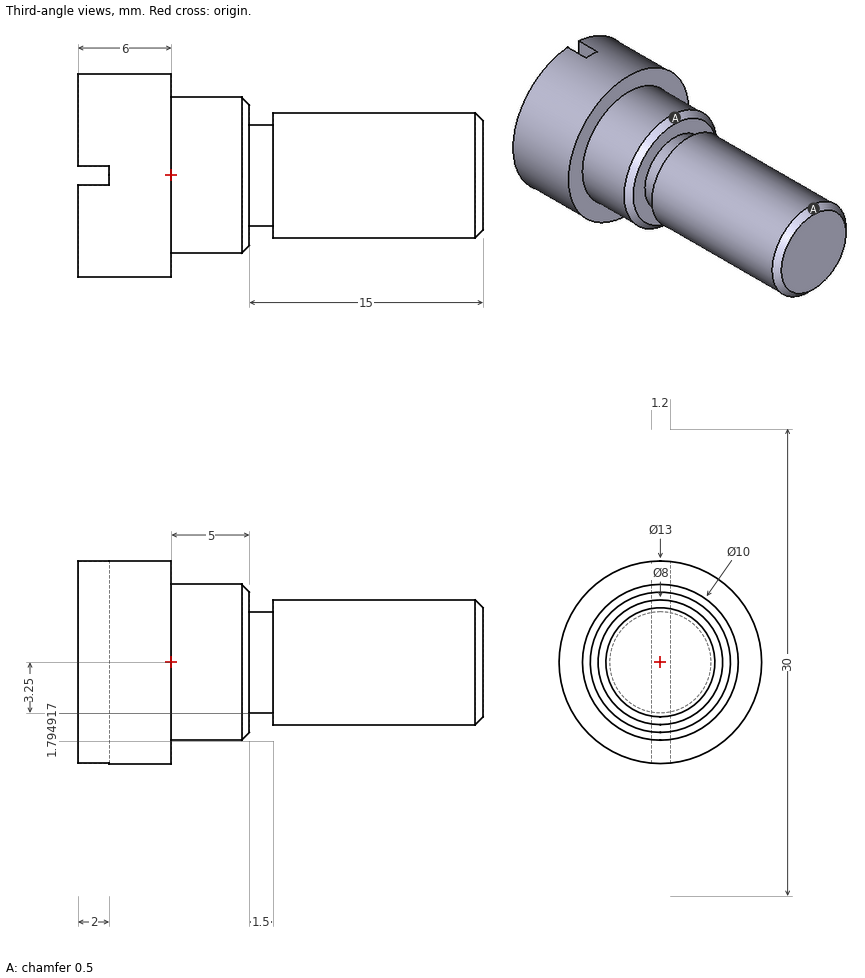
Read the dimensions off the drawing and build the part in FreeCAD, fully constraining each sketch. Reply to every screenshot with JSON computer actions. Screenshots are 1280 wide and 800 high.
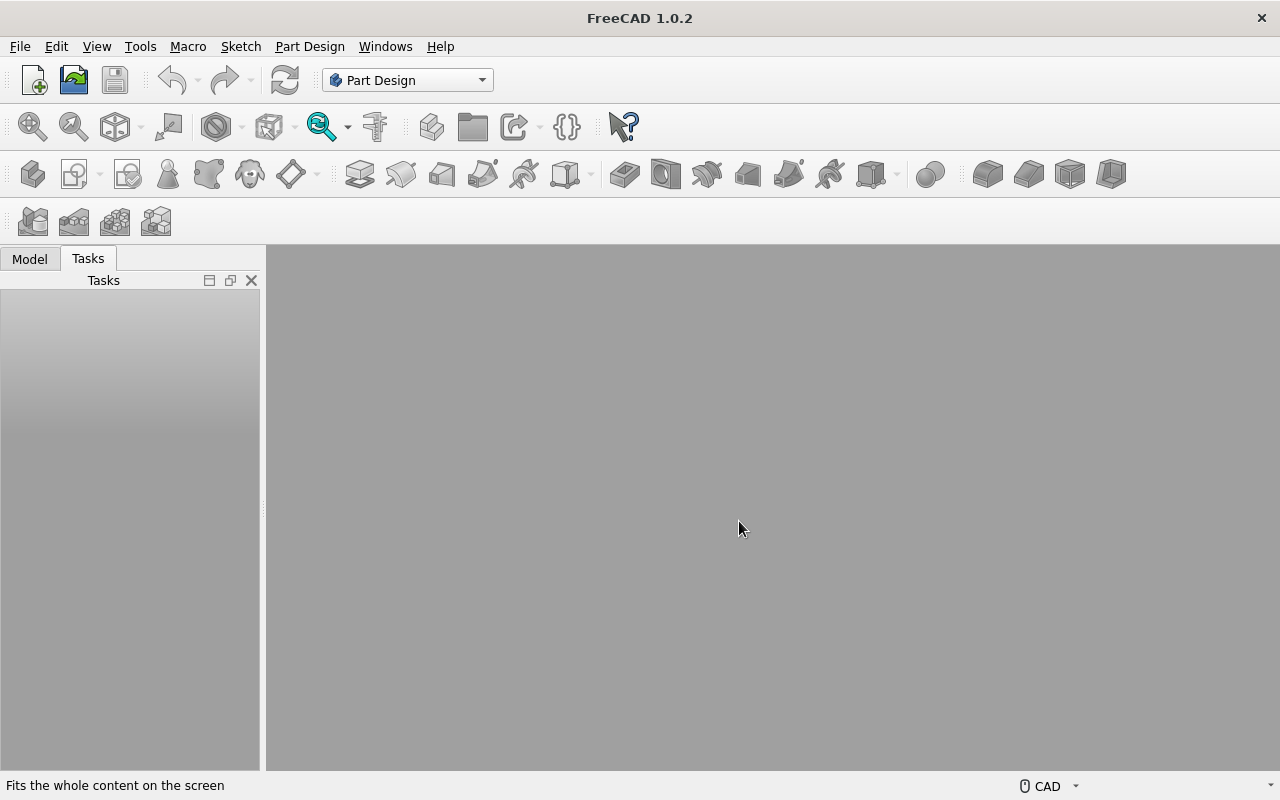
{"action": "left_click", "coordinate": [33, 80]}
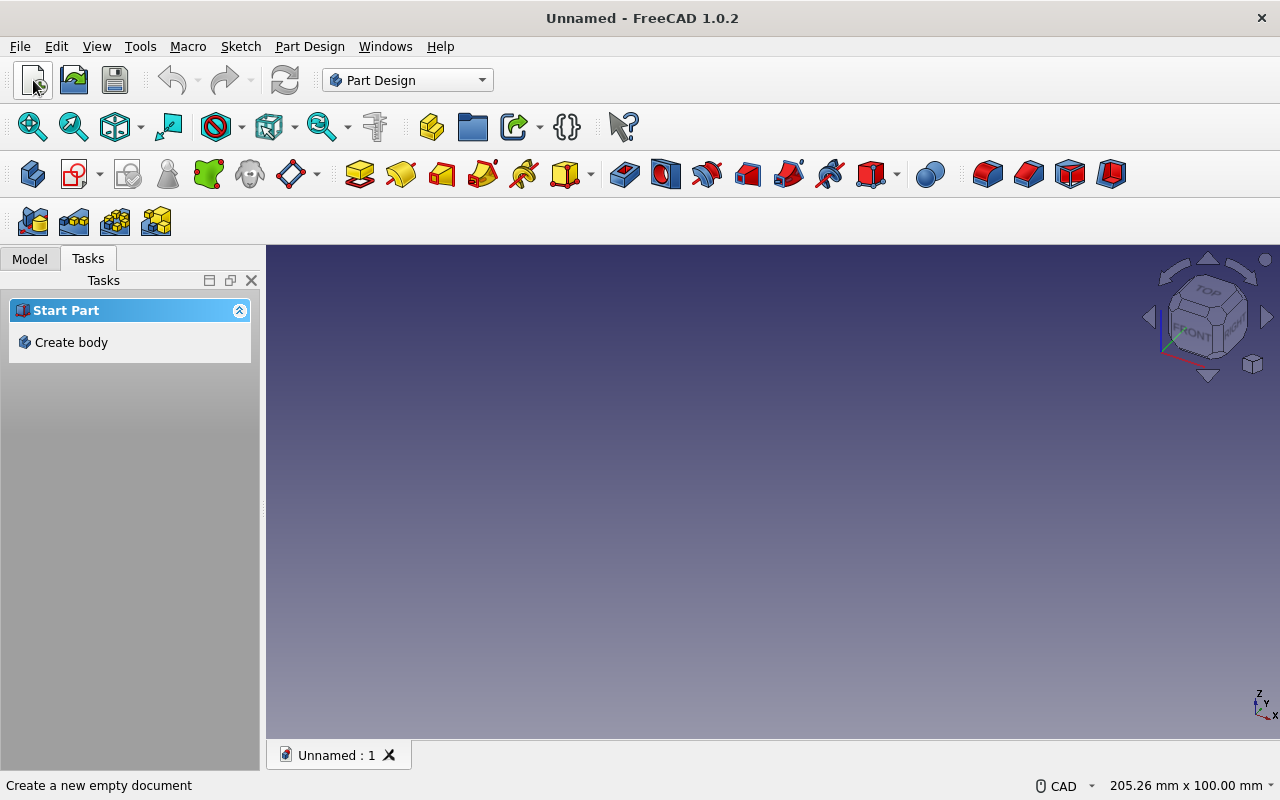
{"action": "left_click", "coordinate": [74, 174]}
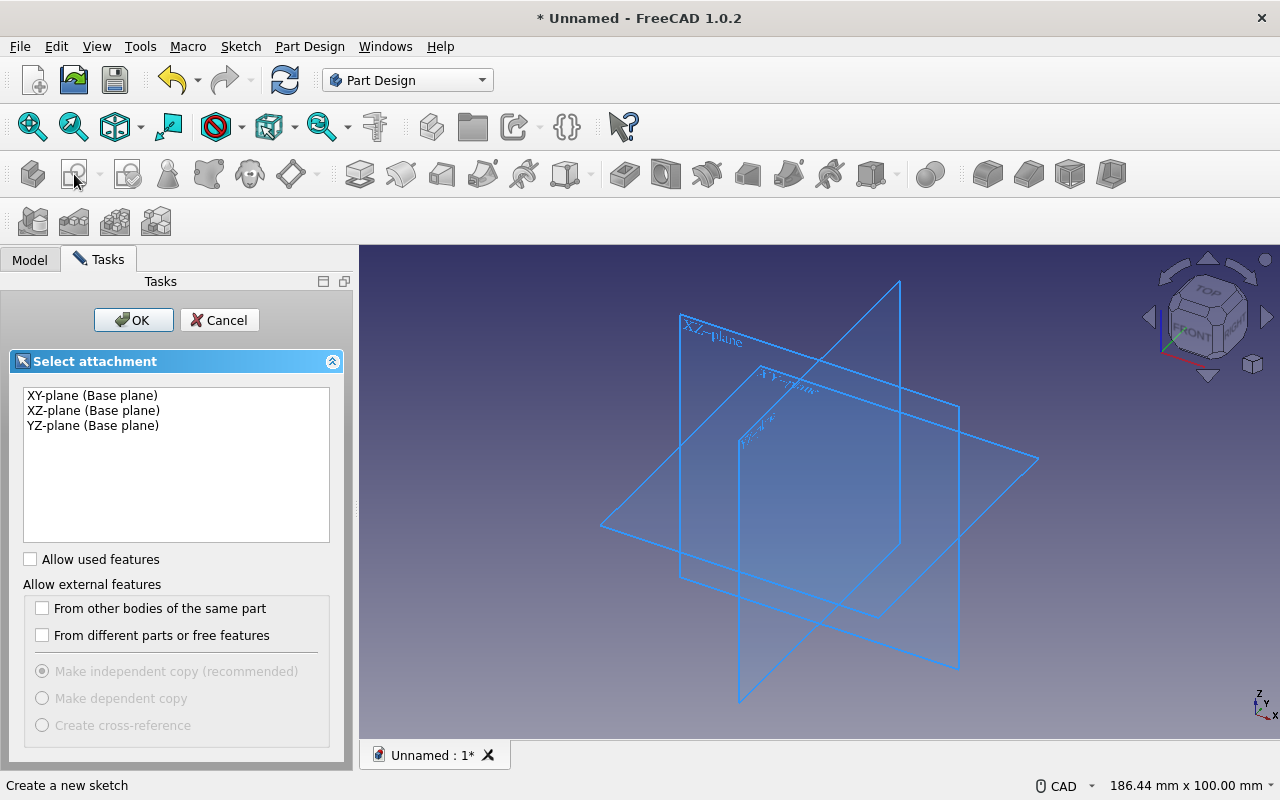
{"action": "left_click", "coordinate": [84, 426]}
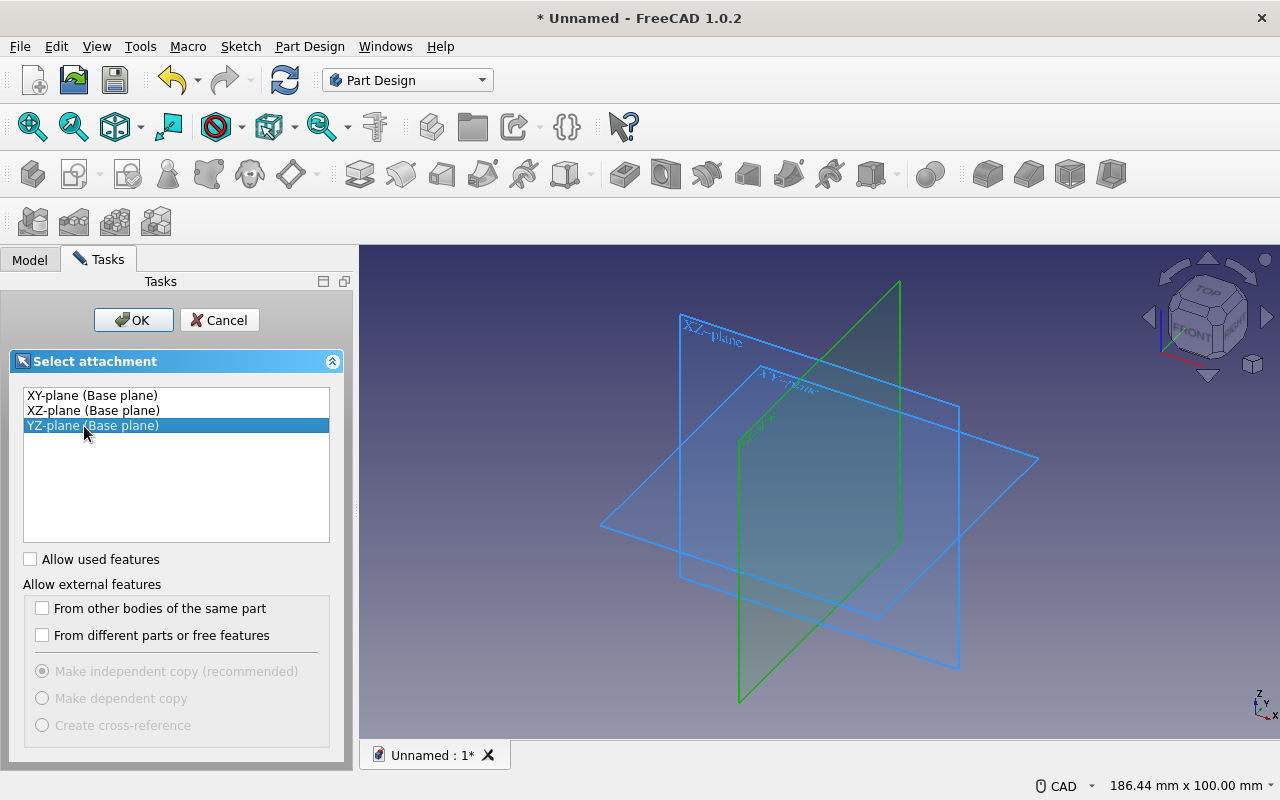
{"action": "left_click", "coordinate": [134, 320]}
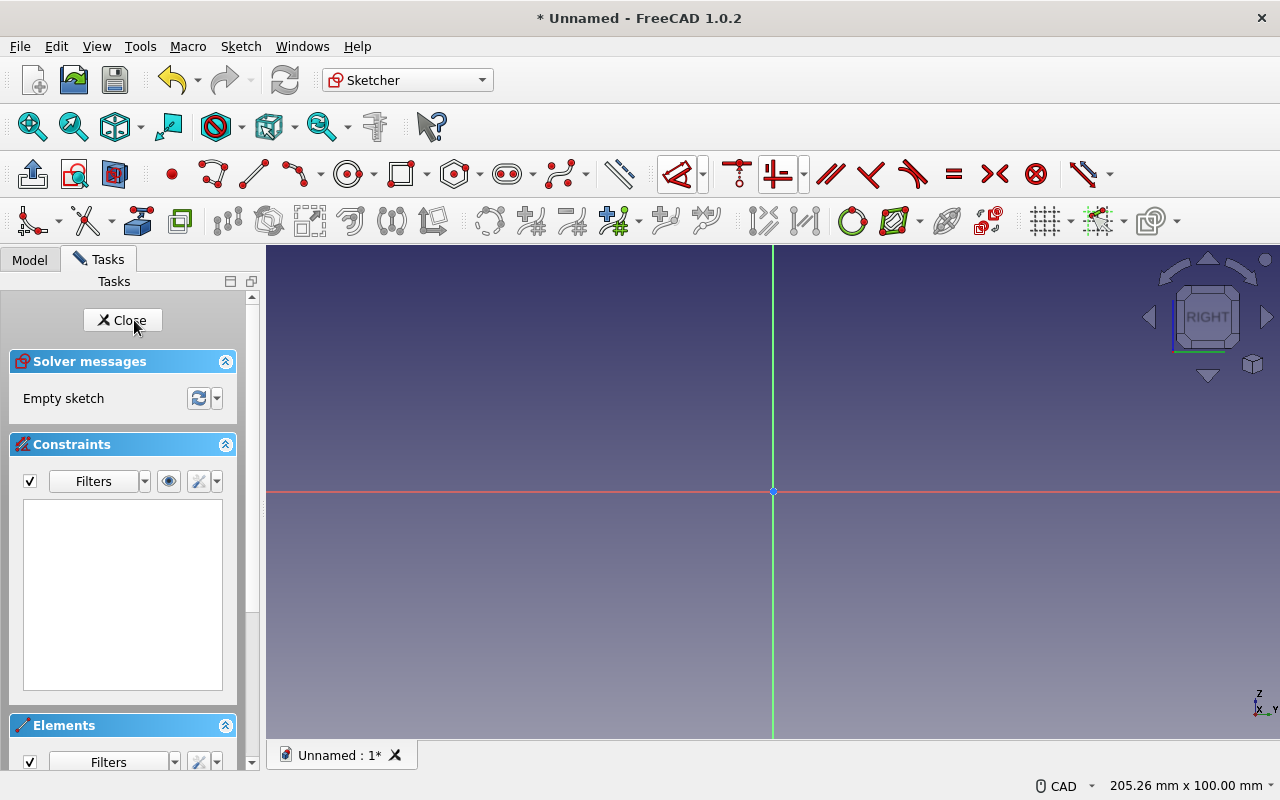
{"action": "scroll", "coordinate": [787, 492], "scroll_direction": "up", "scroll_amount": 9}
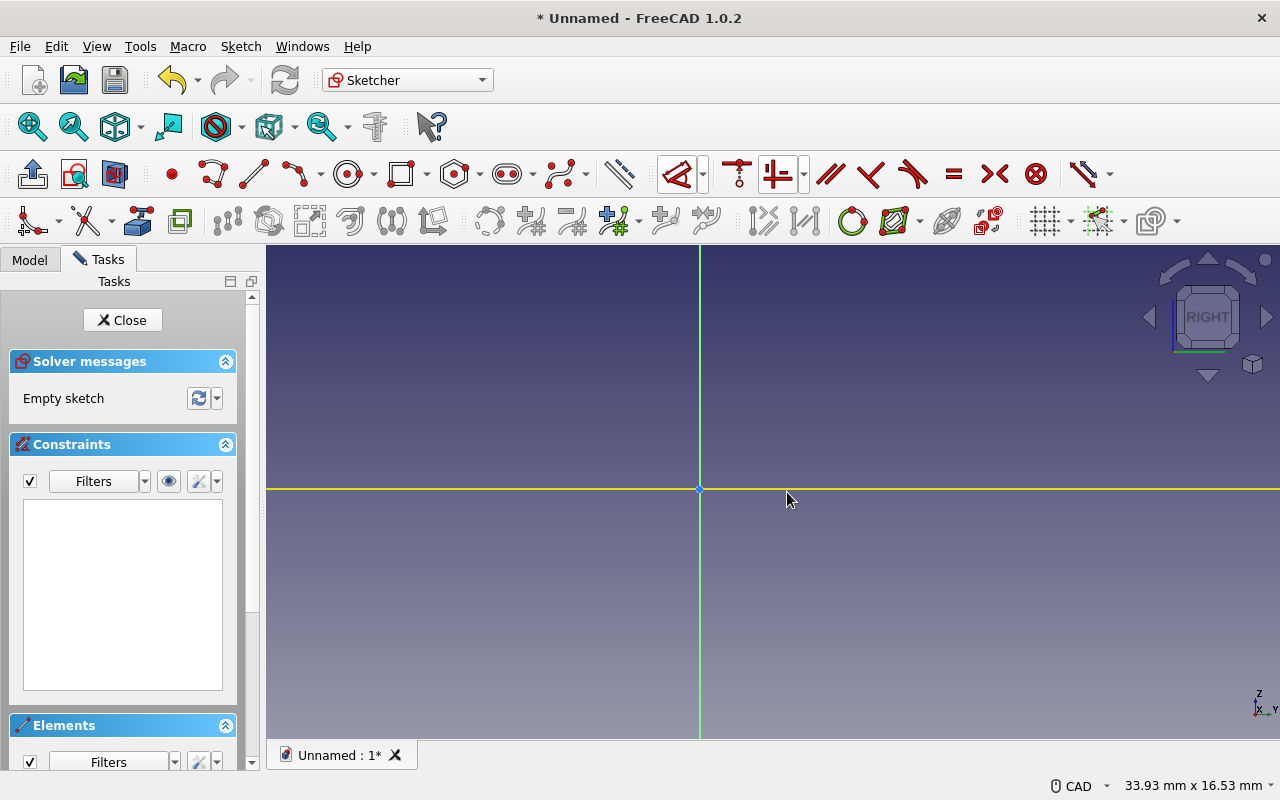
{"action": "left_click", "coordinate": [348, 174]}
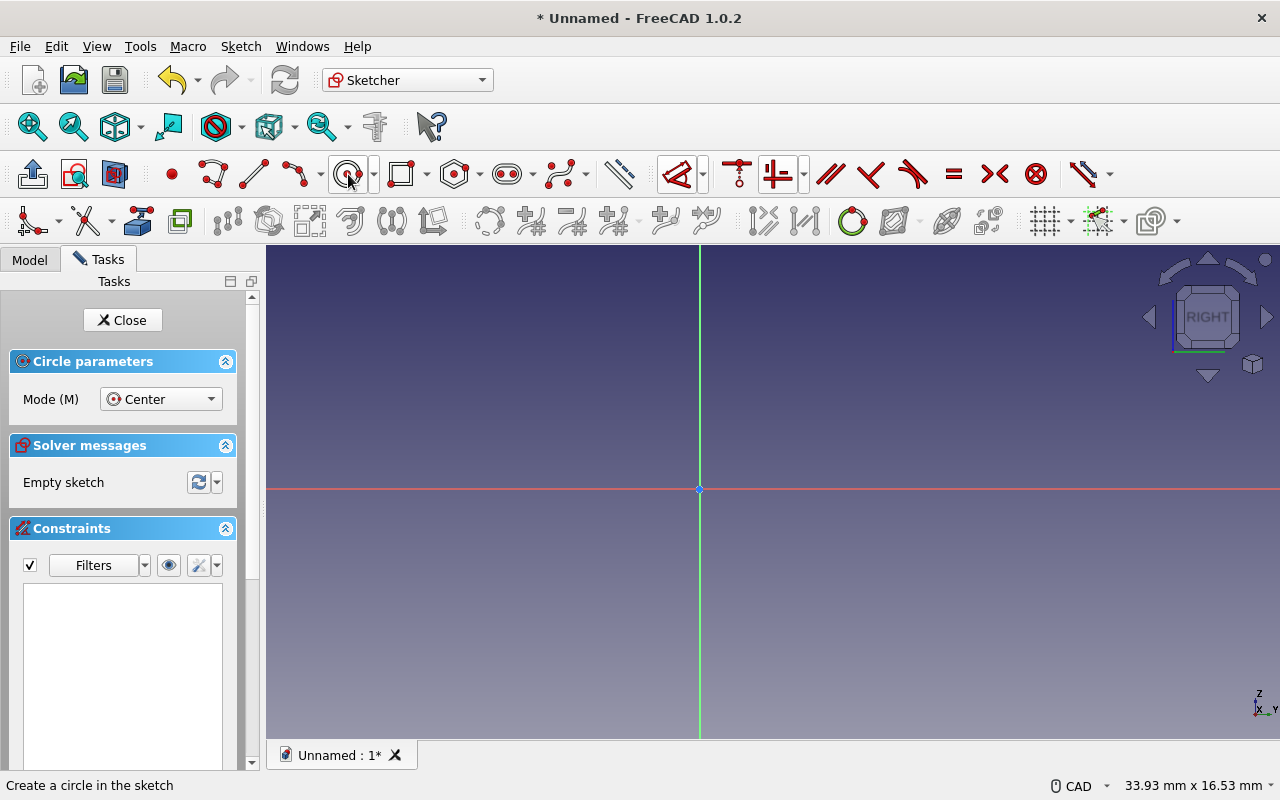
{"action": "left_click", "coordinate": [700, 489]}
{"action": "mouse_move", "coordinate": [805, 384]}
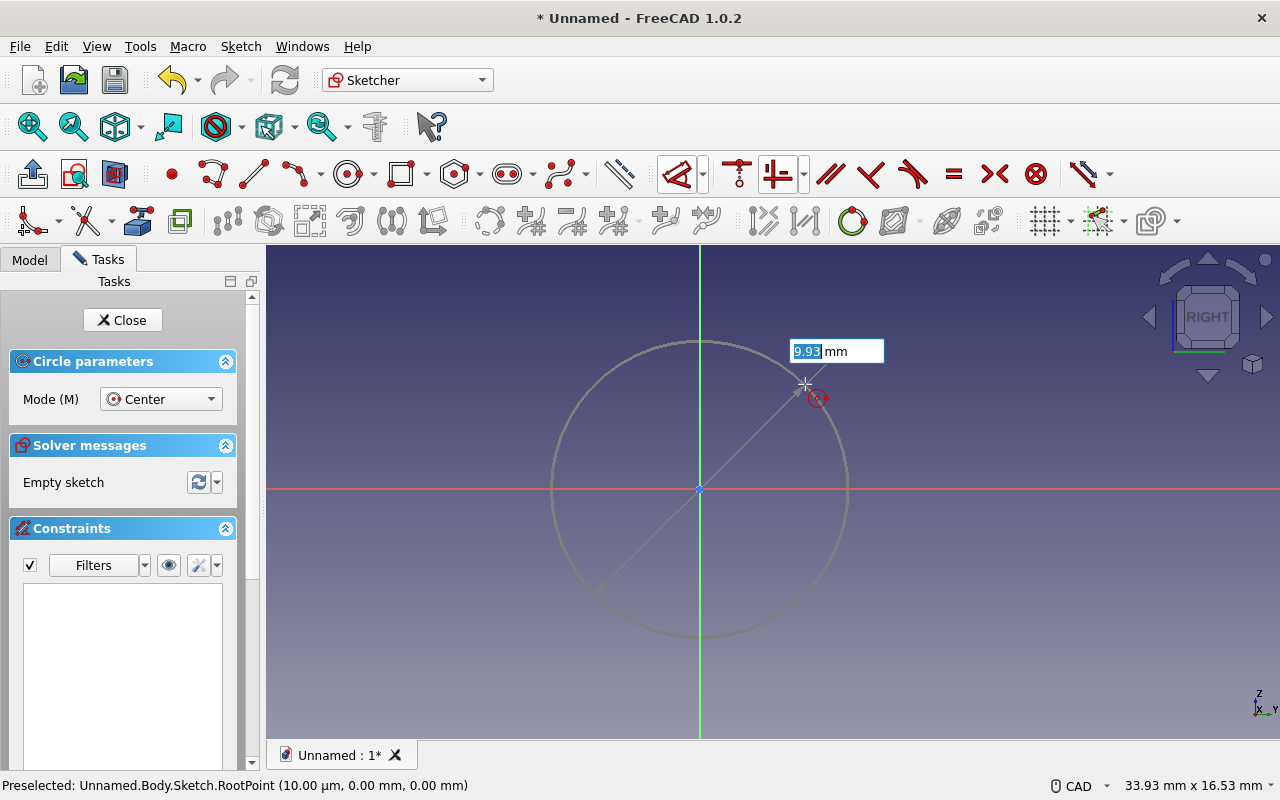
{"action": "type", "text": "10"}
{"action": "key", "text": "Return"}
{"action": "key", "text": "Escape"}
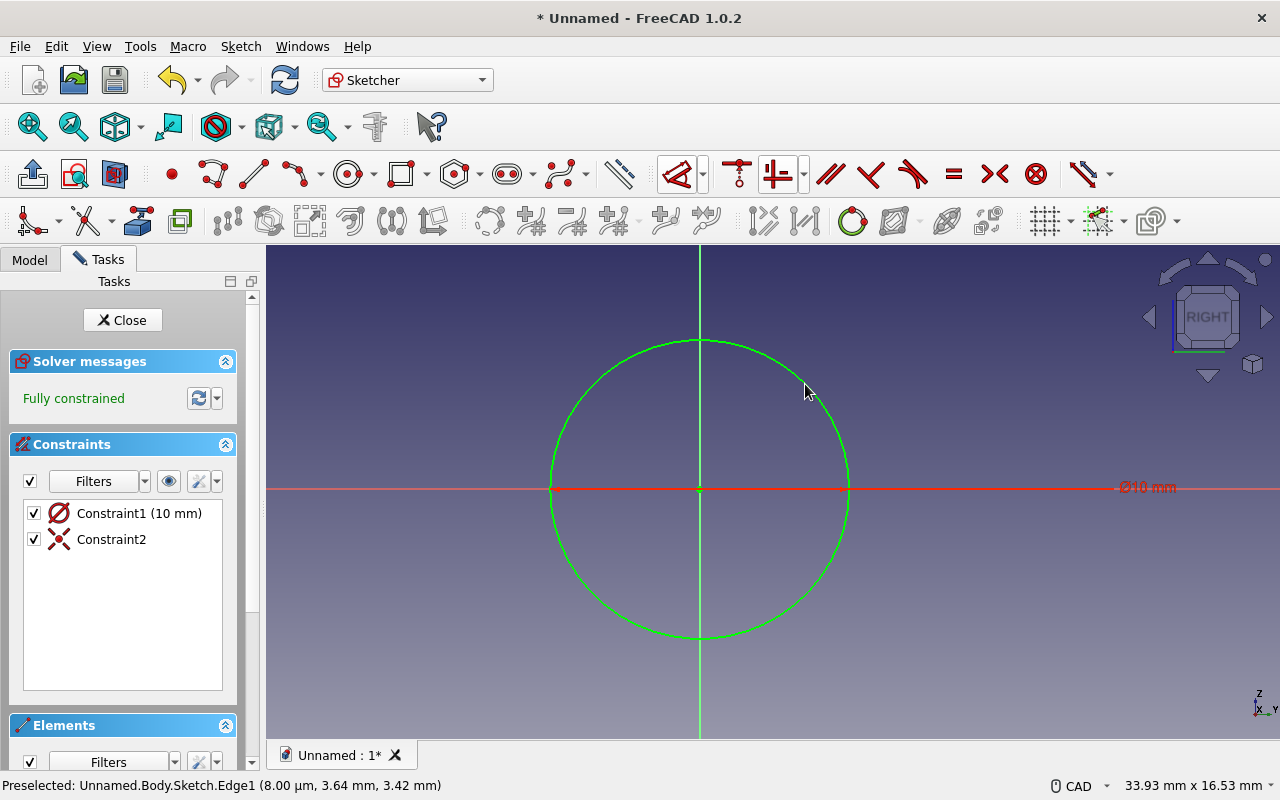
{"action": "left_click", "coordinate": [123, 320]}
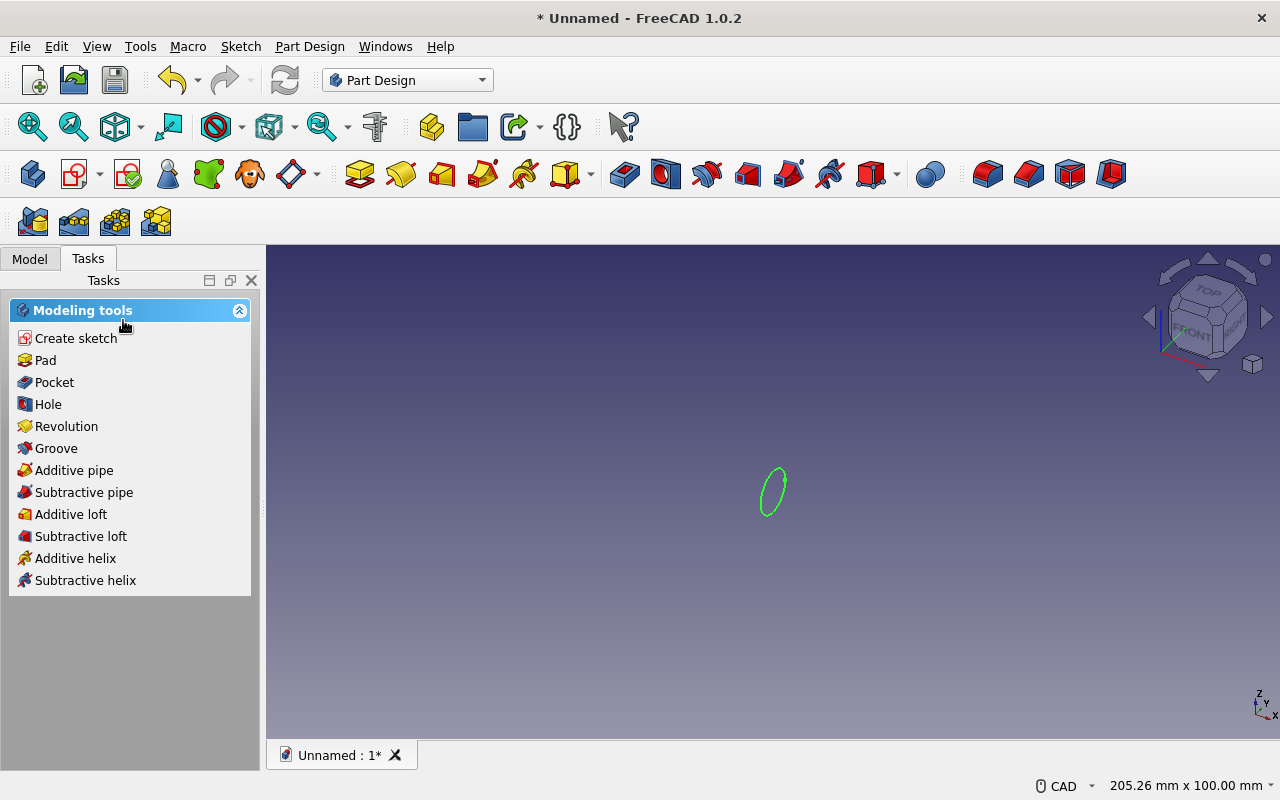
{"action": "left_click", "coordinate": [360, 174]}